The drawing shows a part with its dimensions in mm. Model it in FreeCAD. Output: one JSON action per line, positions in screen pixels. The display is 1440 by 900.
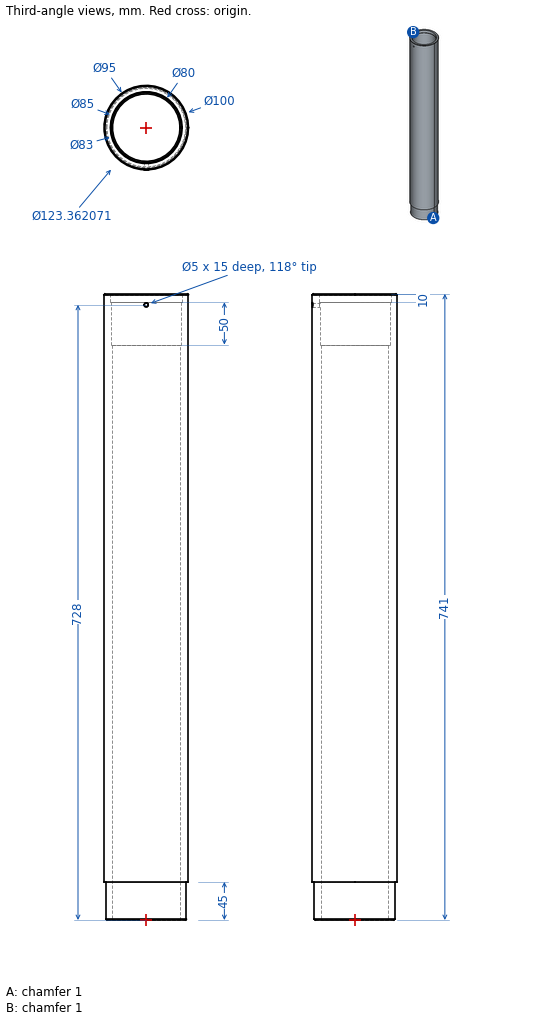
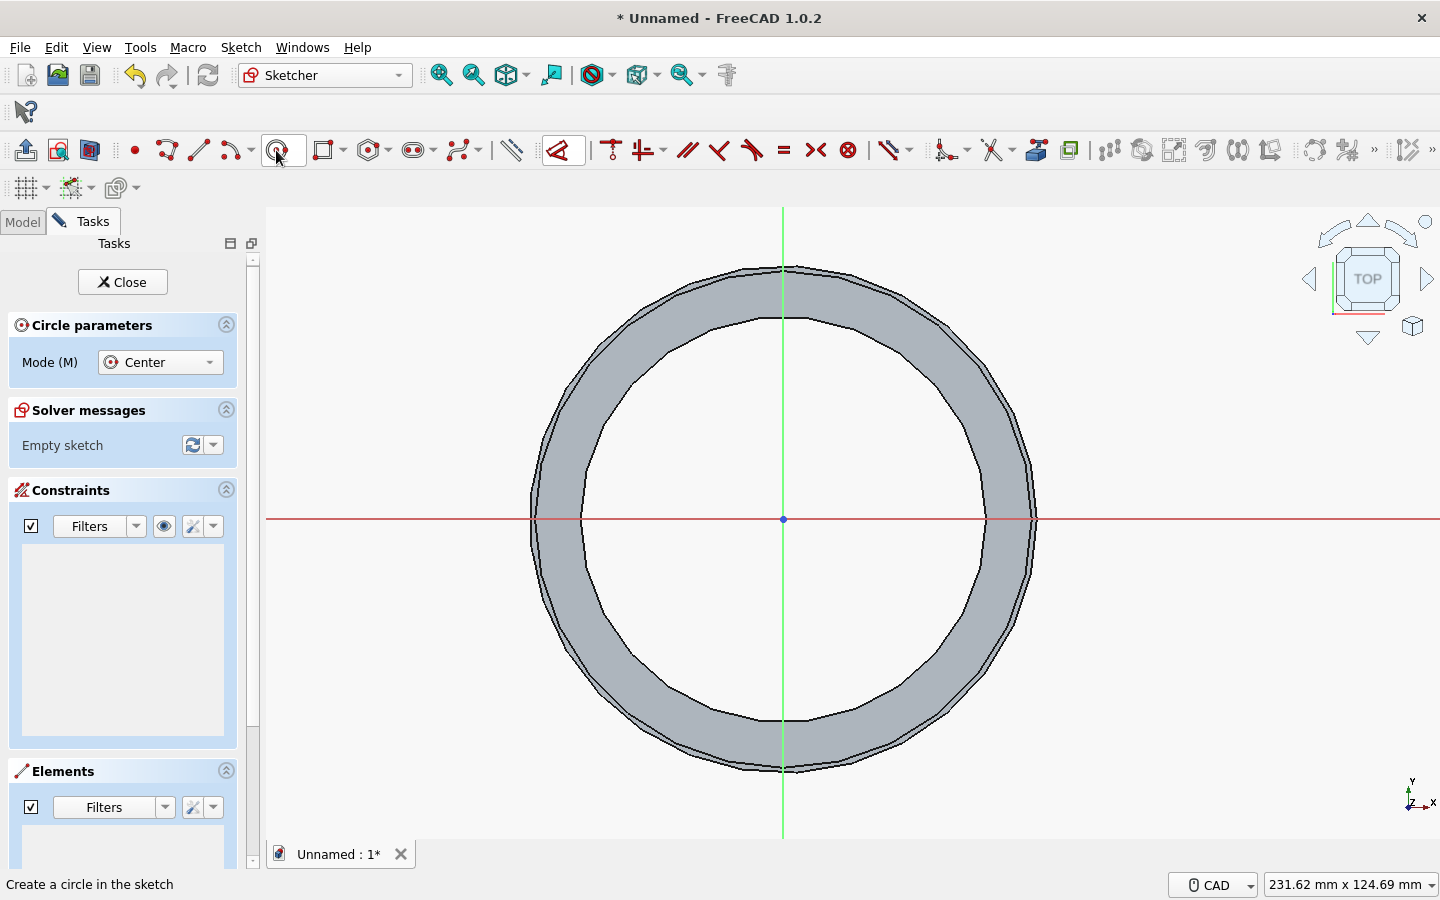
{"action": "left_click", "coordinate": [783, 519]}
{"action": "left_click", "coordinate": [936, 367]}
{"action": "key", "text": "Escape"}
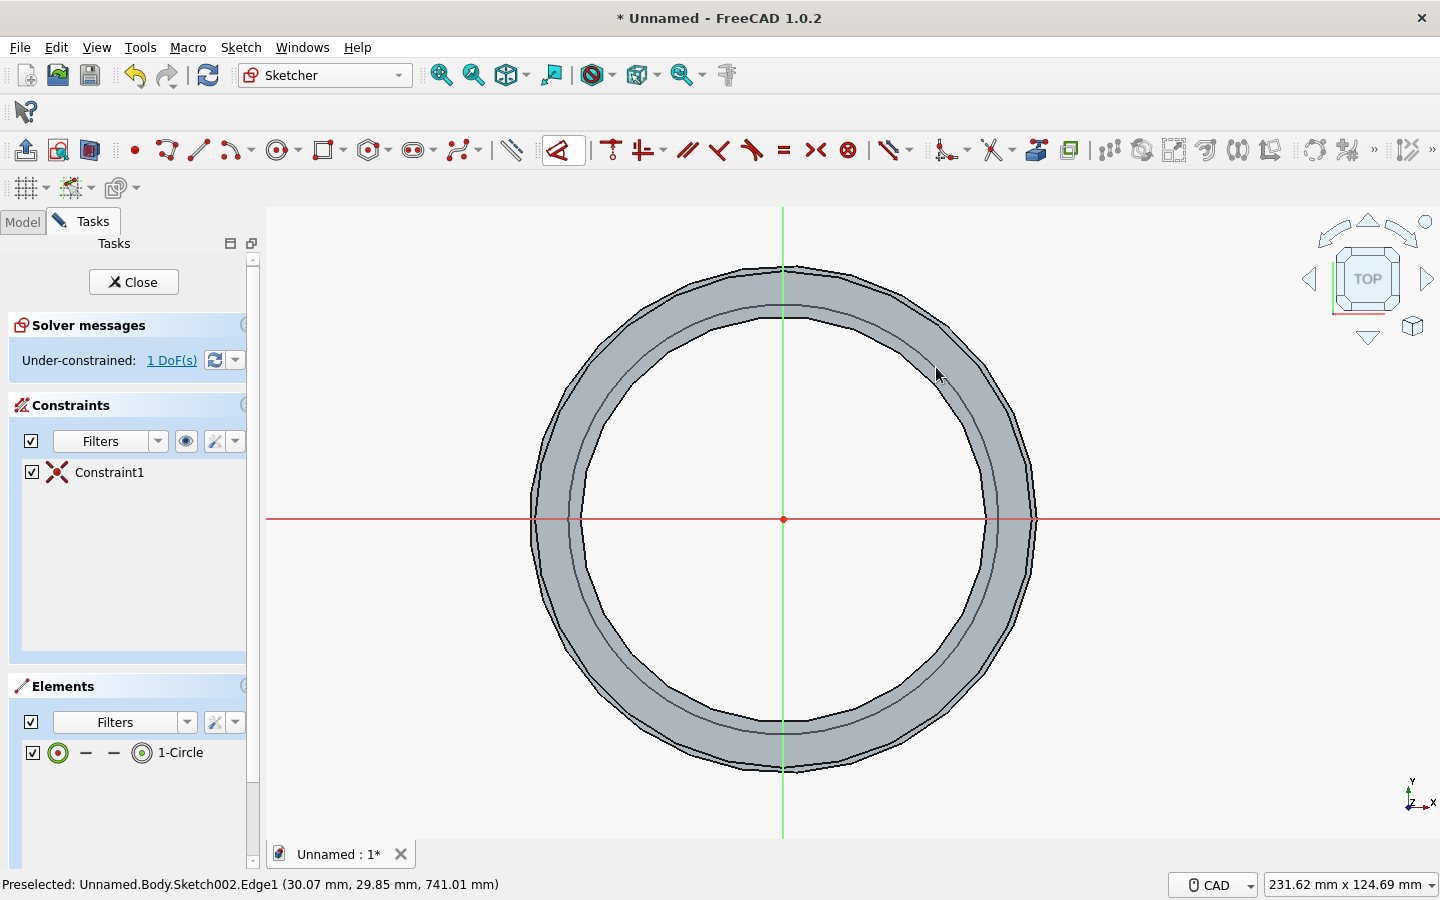
{"action": "left_click", "coordinate": [935, 367]}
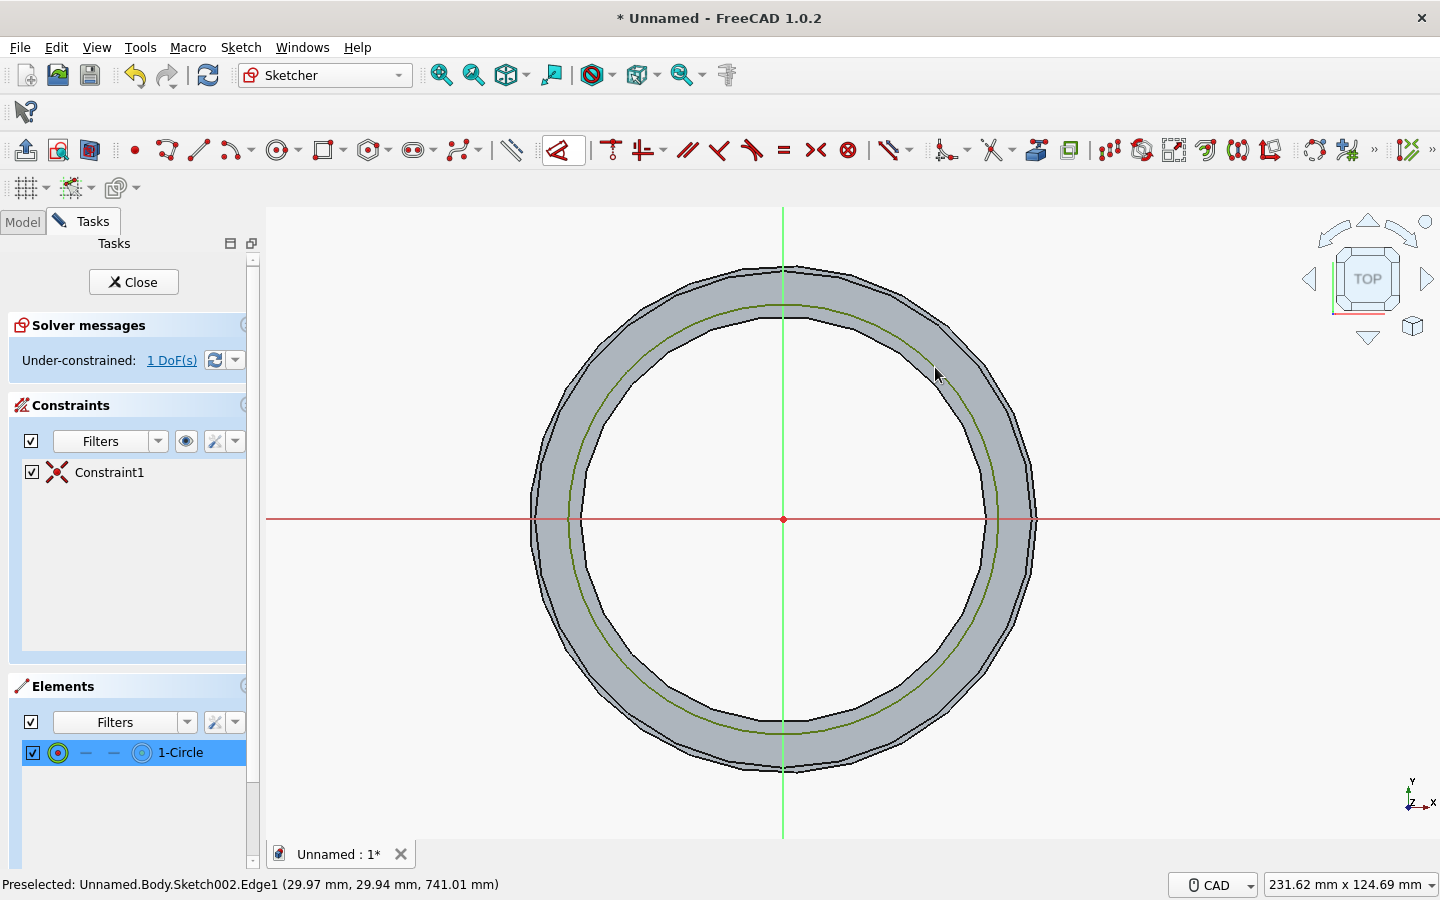
{"action": "key", "text": "k o"}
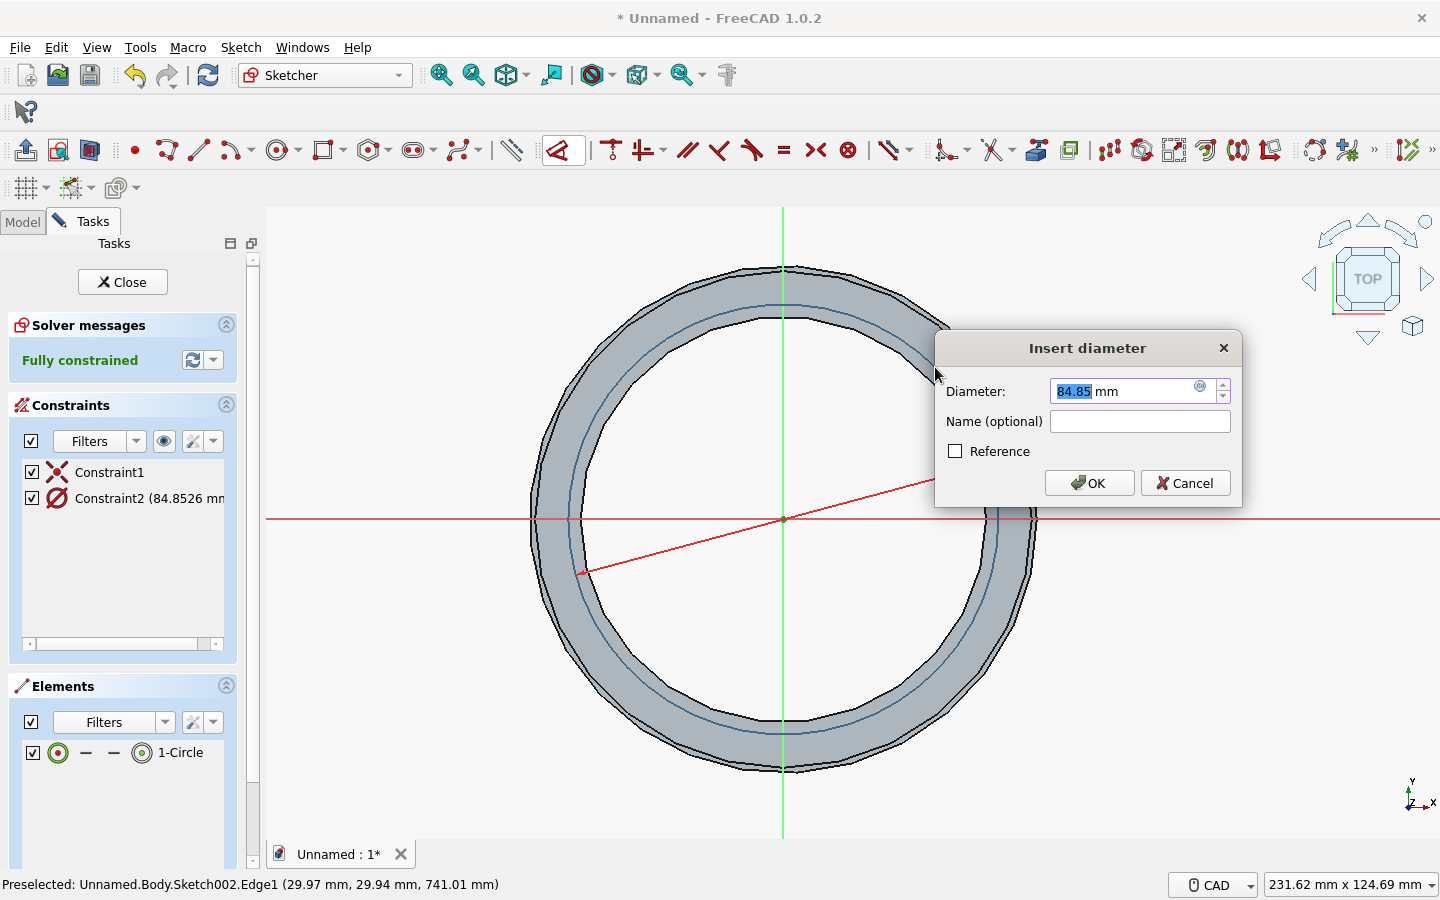
{"action": "type", "text": "85"}
{"action": "key", "text": "Return"}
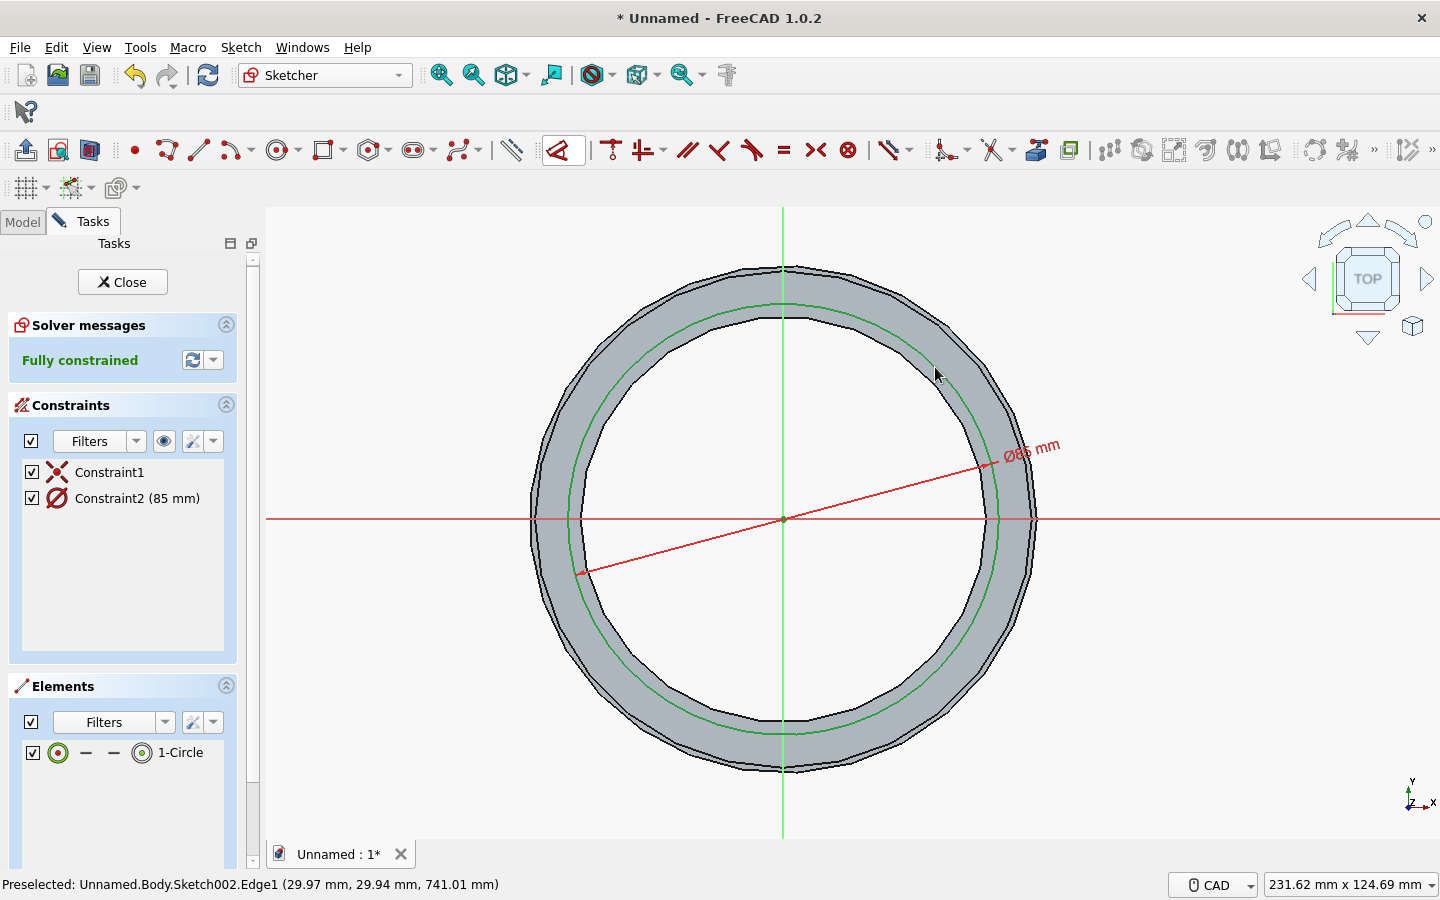
{"action": "left_click", "coordinate": [123, 282]}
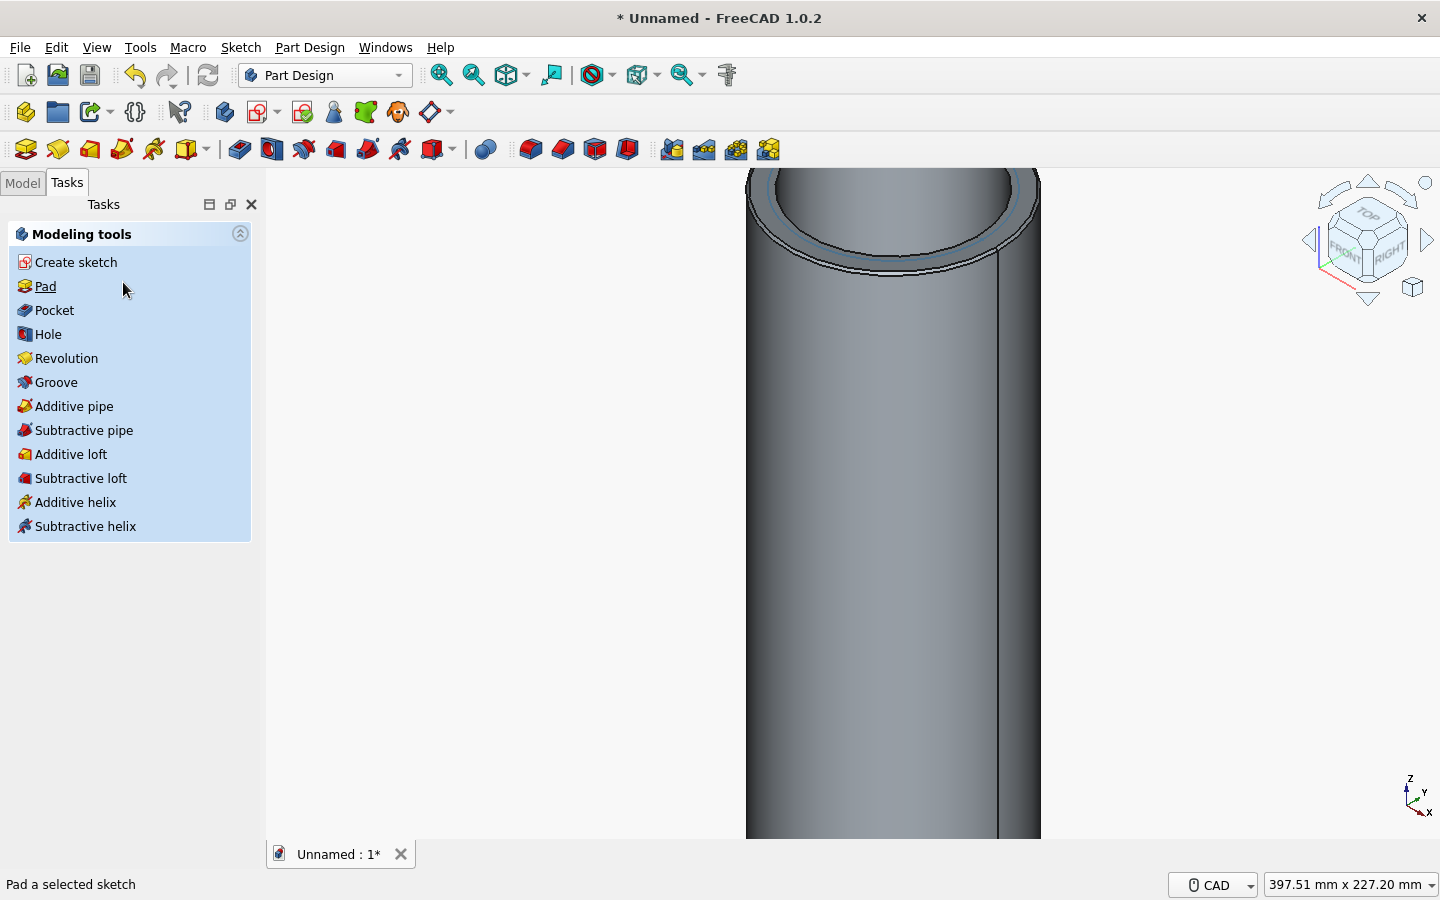
{"action": "left_click", "coordinate": [240, 150]}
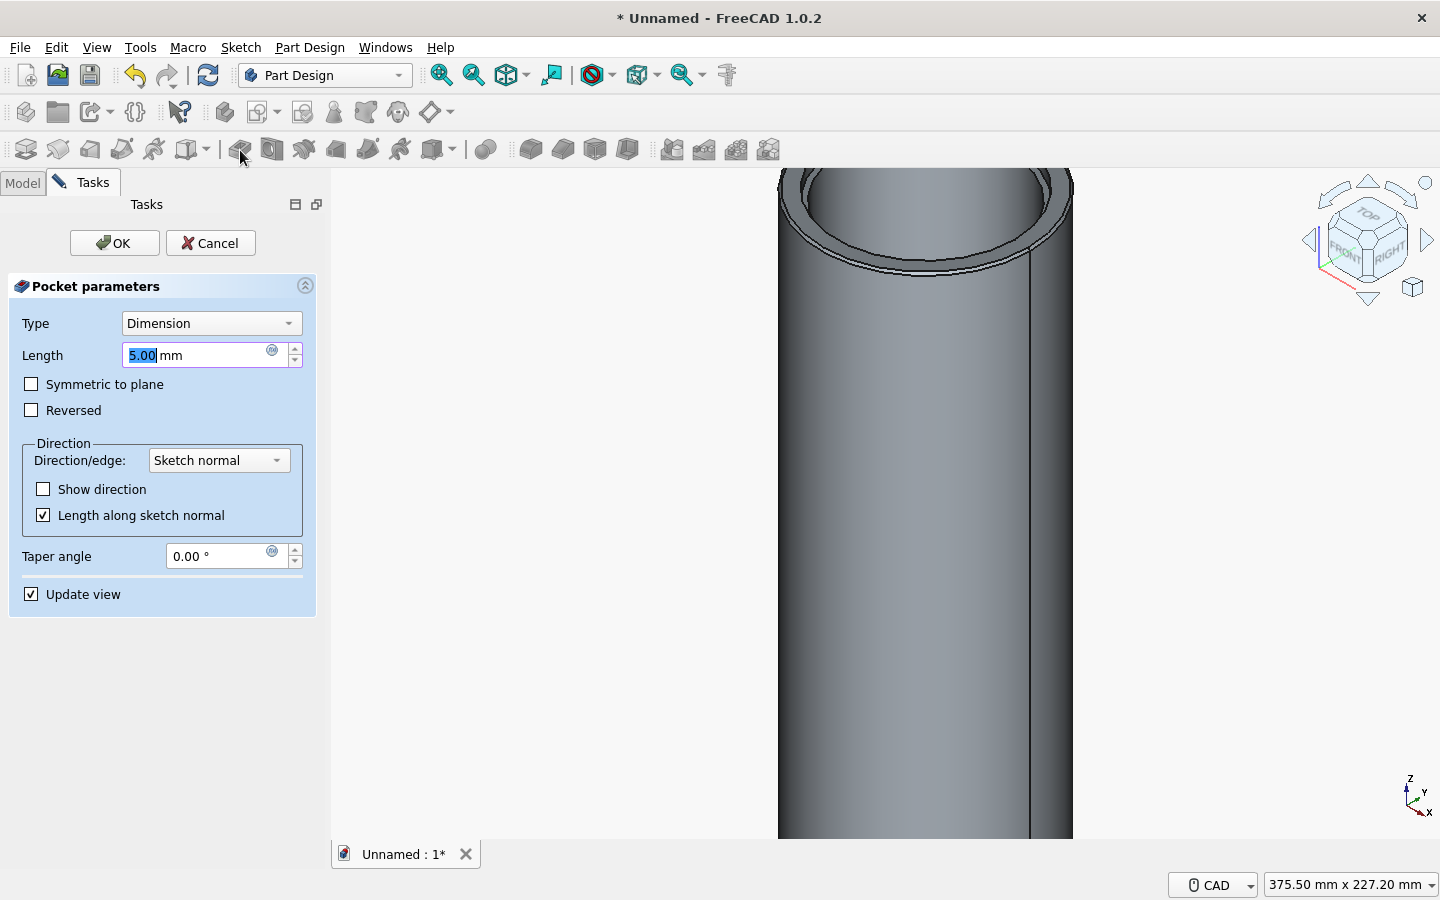
{"action": "type", "text": "10"}
{"action": "key", "text": "Tab"}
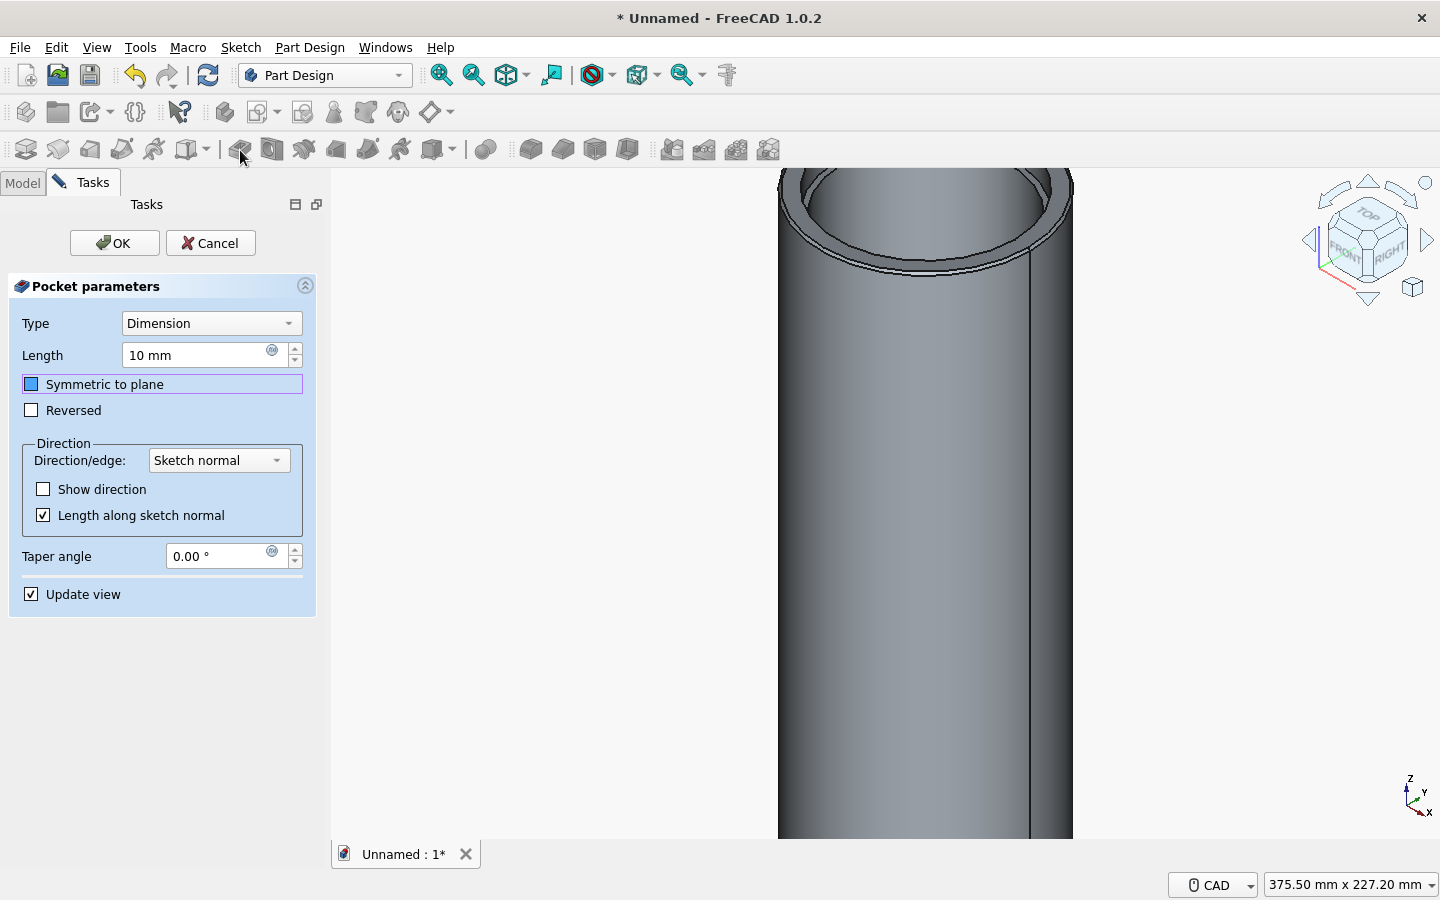
{"action": "left_click", "coordinate": [115, 243]}